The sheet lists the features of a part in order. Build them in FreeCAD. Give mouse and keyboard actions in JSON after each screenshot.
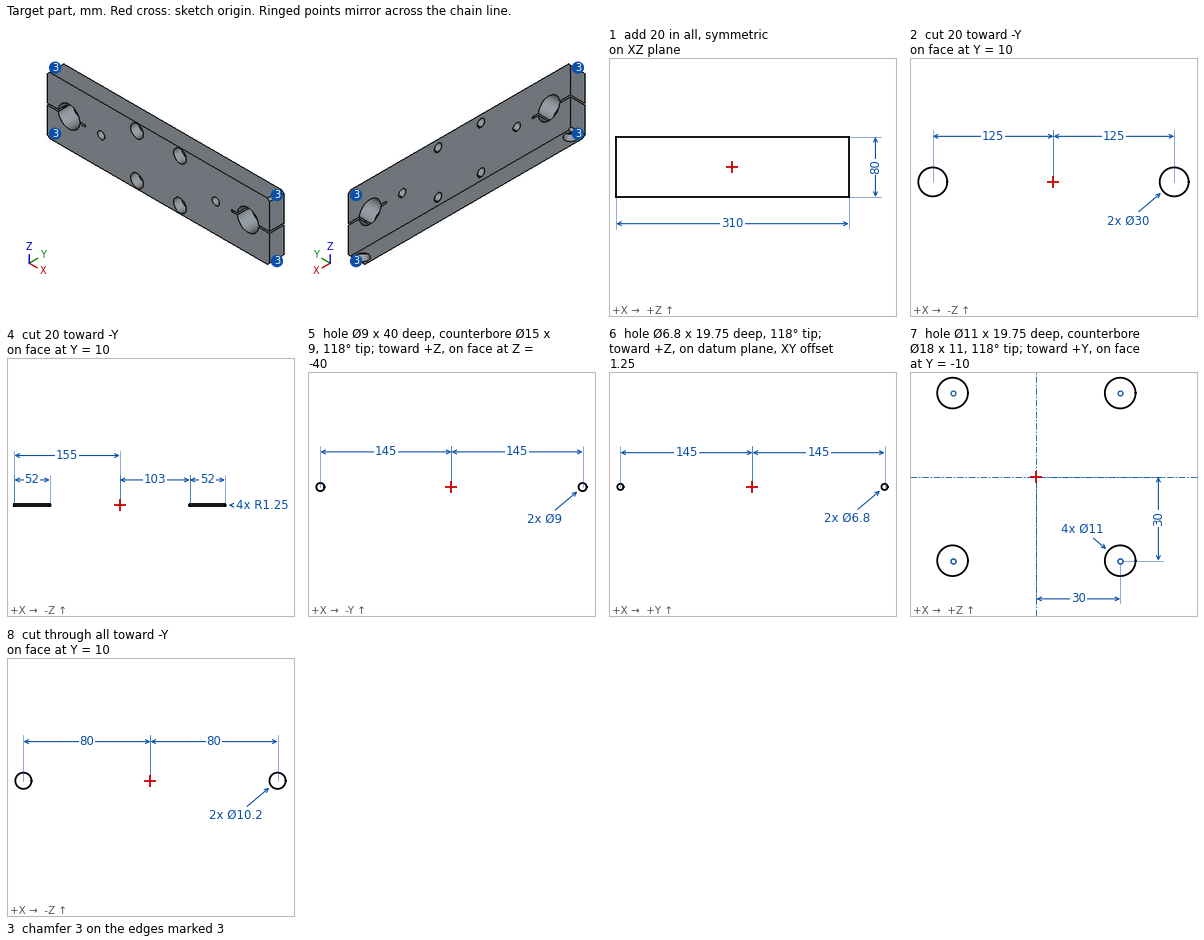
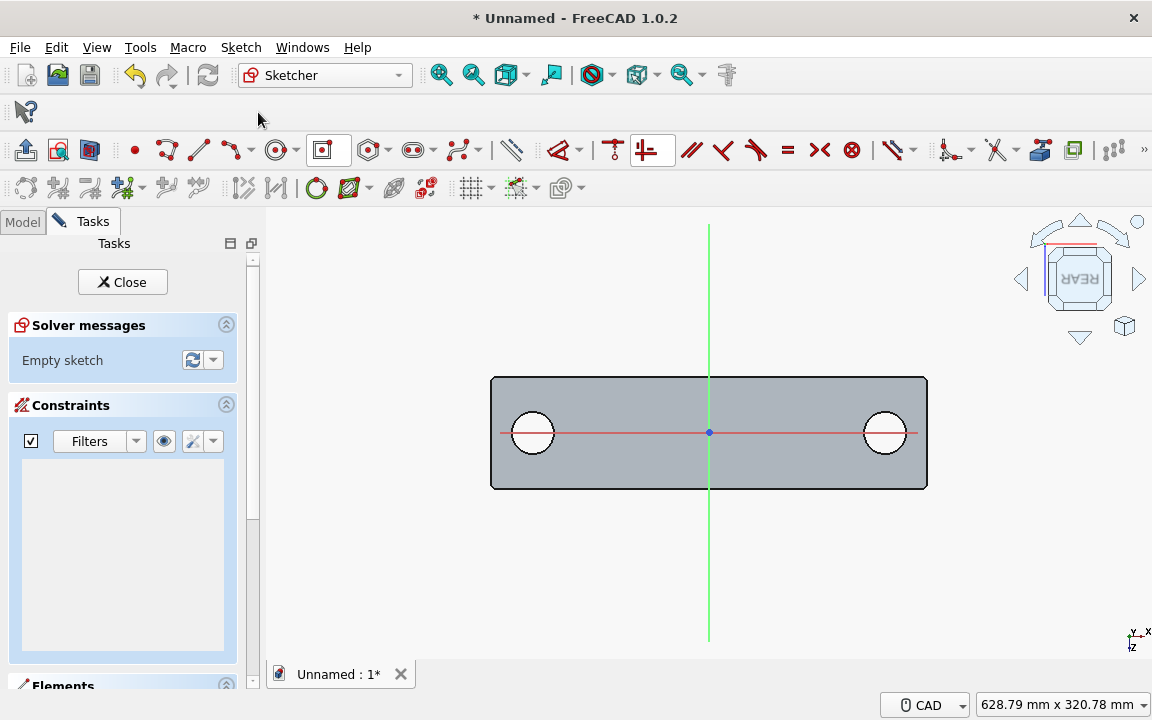
{"action": "left_click", "coordinate": [414, 150]}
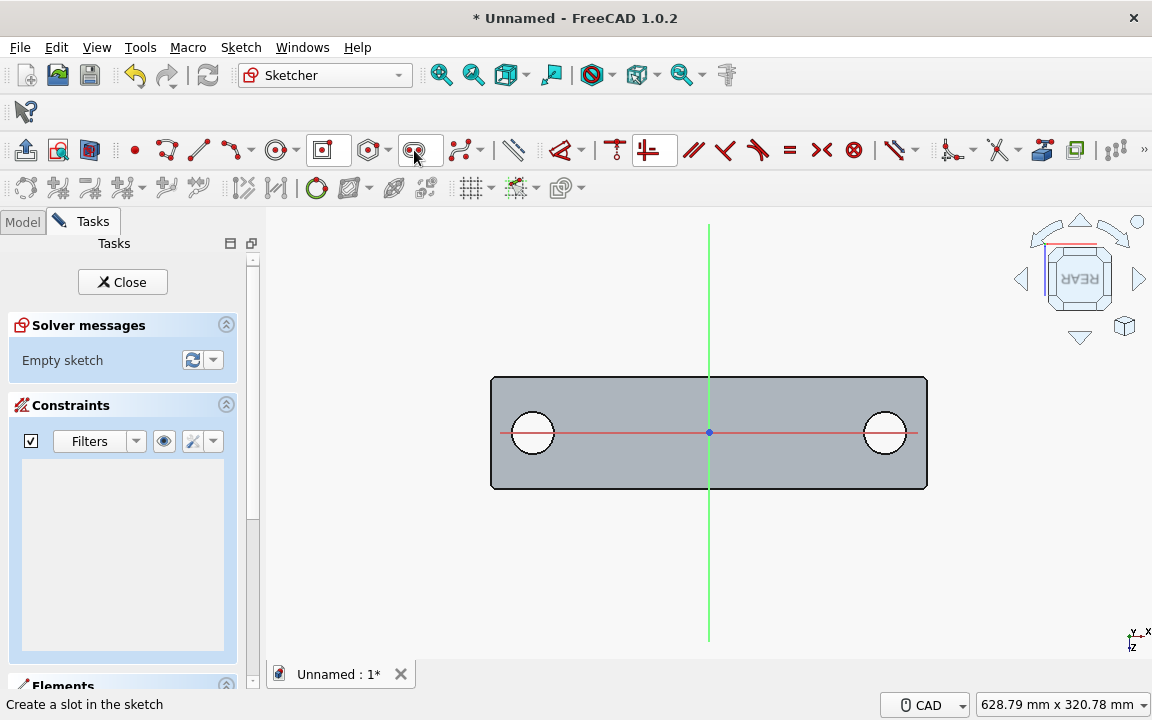
{"action": "scroll", "coordinate": [854, 433], "scroll_direction": "up", "scroll_amount": 13}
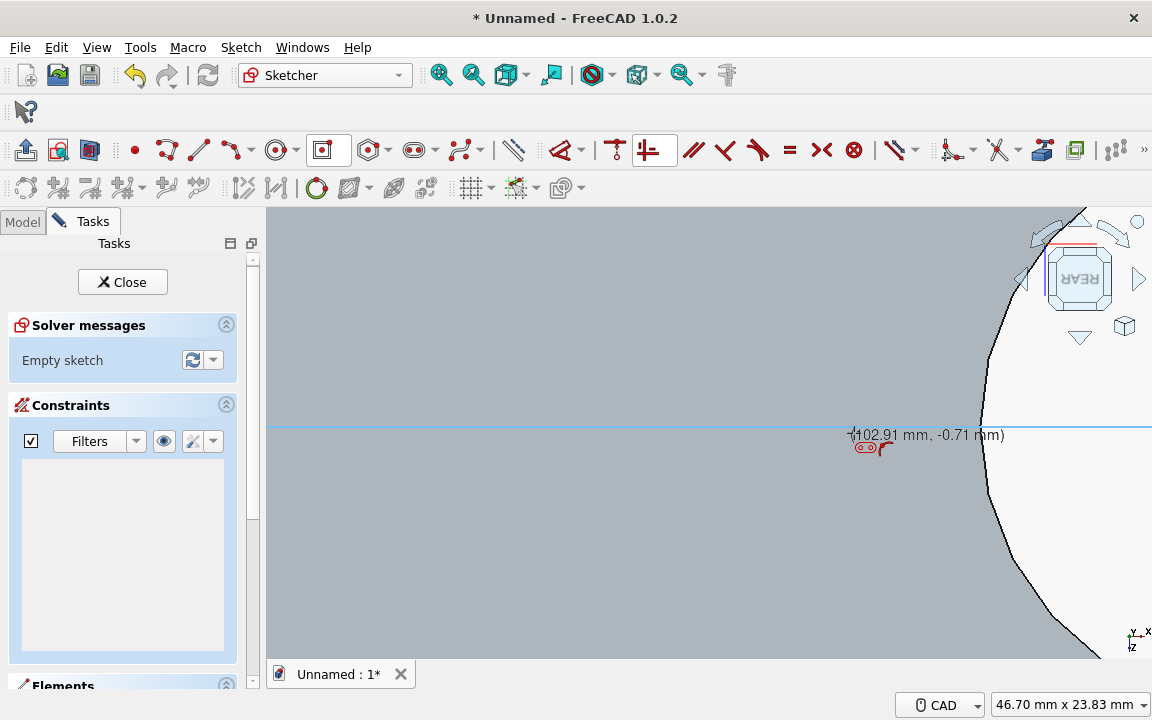
{"action": "scroll", "coordinate": [815, 434], "scroll_direction": "down", "scroll_amount": 12}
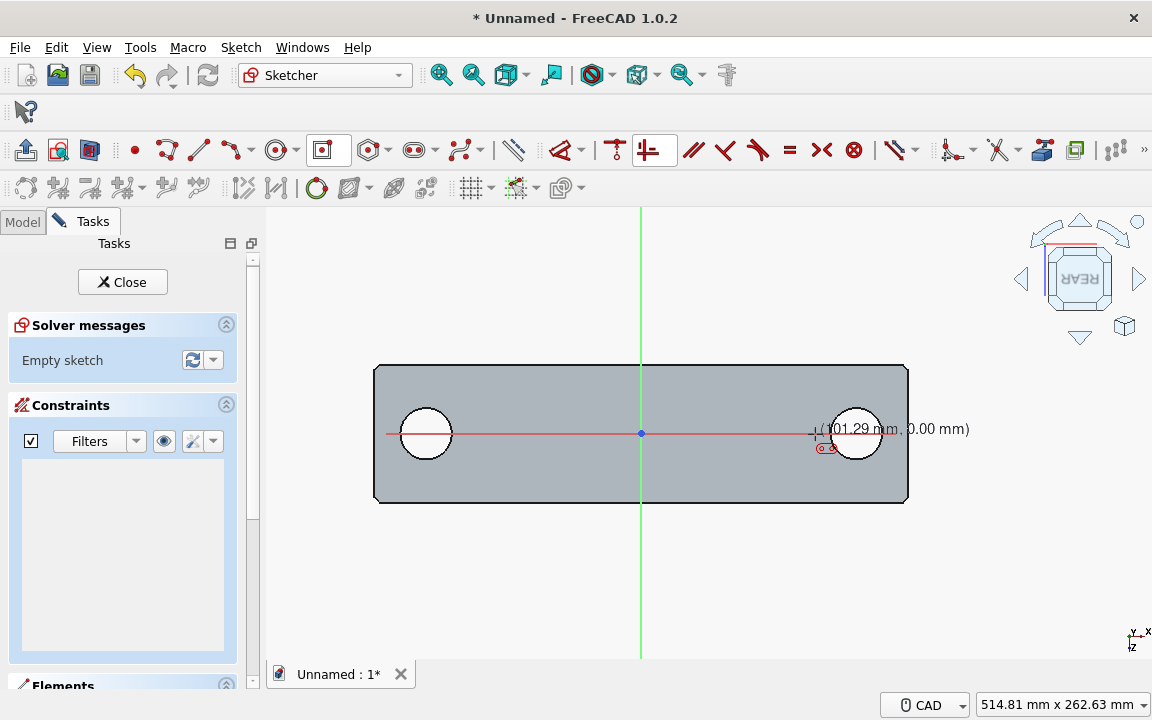
{"action": "left_click", "coordinate": [819, 434]}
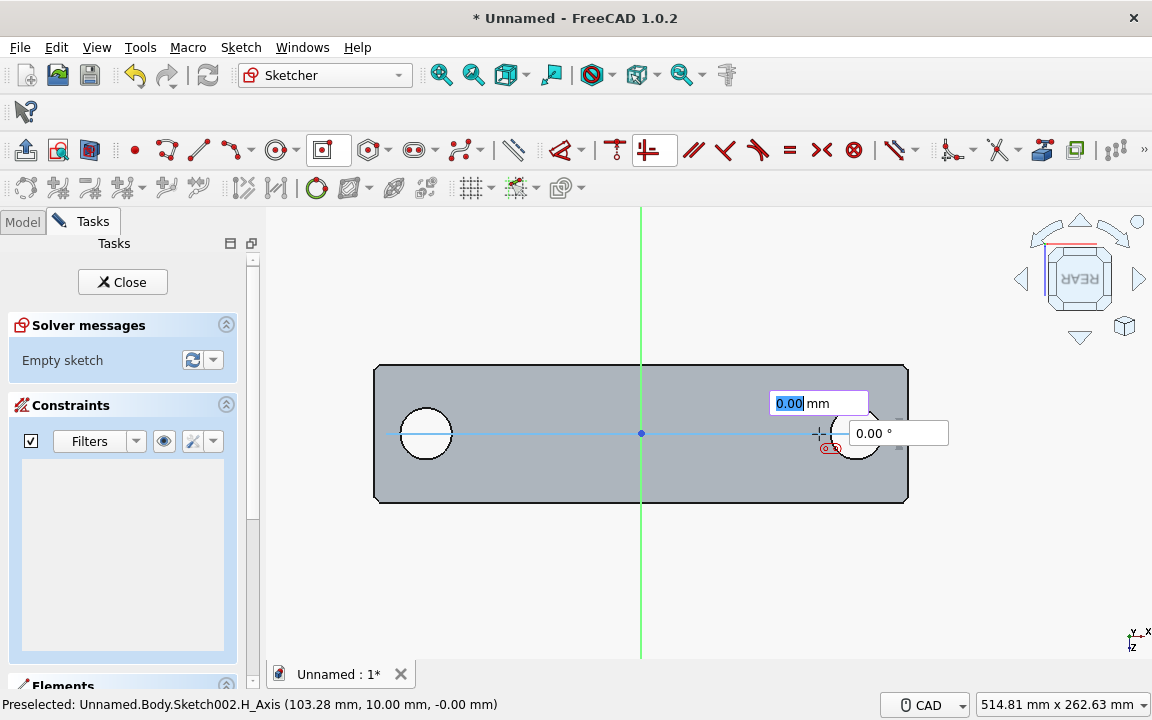
{"action": "left_click", "coordinate": [908, 425]}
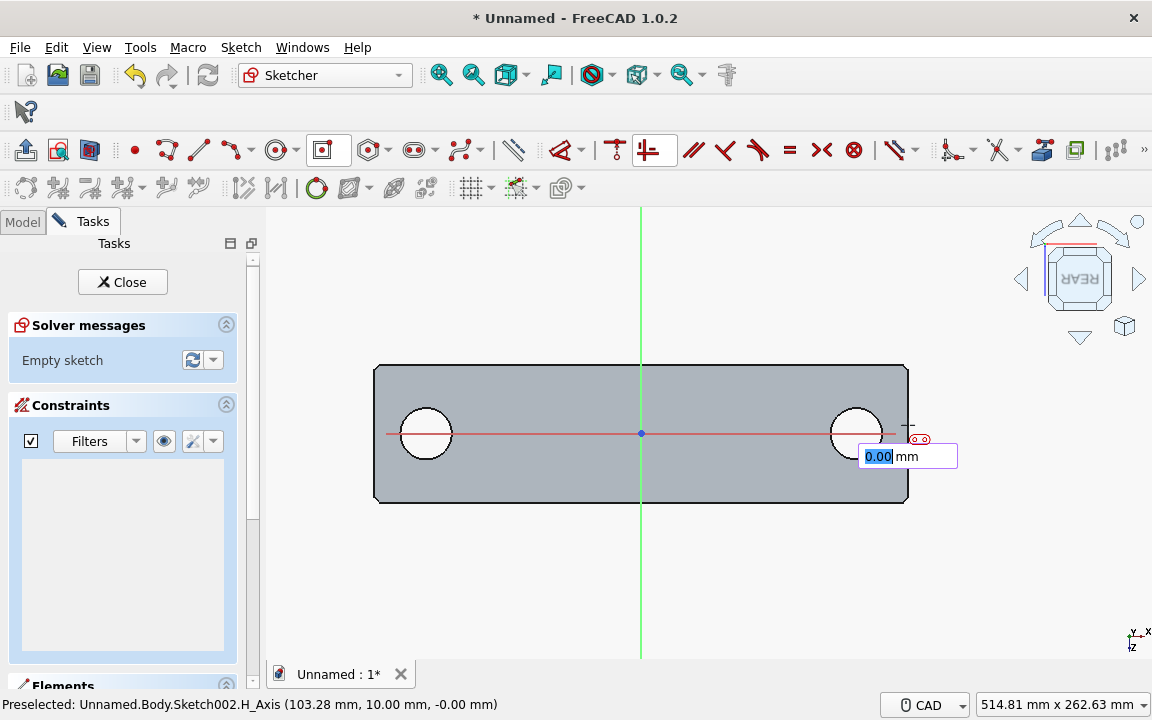
{"action": "scroll", "coordinate": [863, 436], "scroll_direction": "up", "scroll_amount": 10}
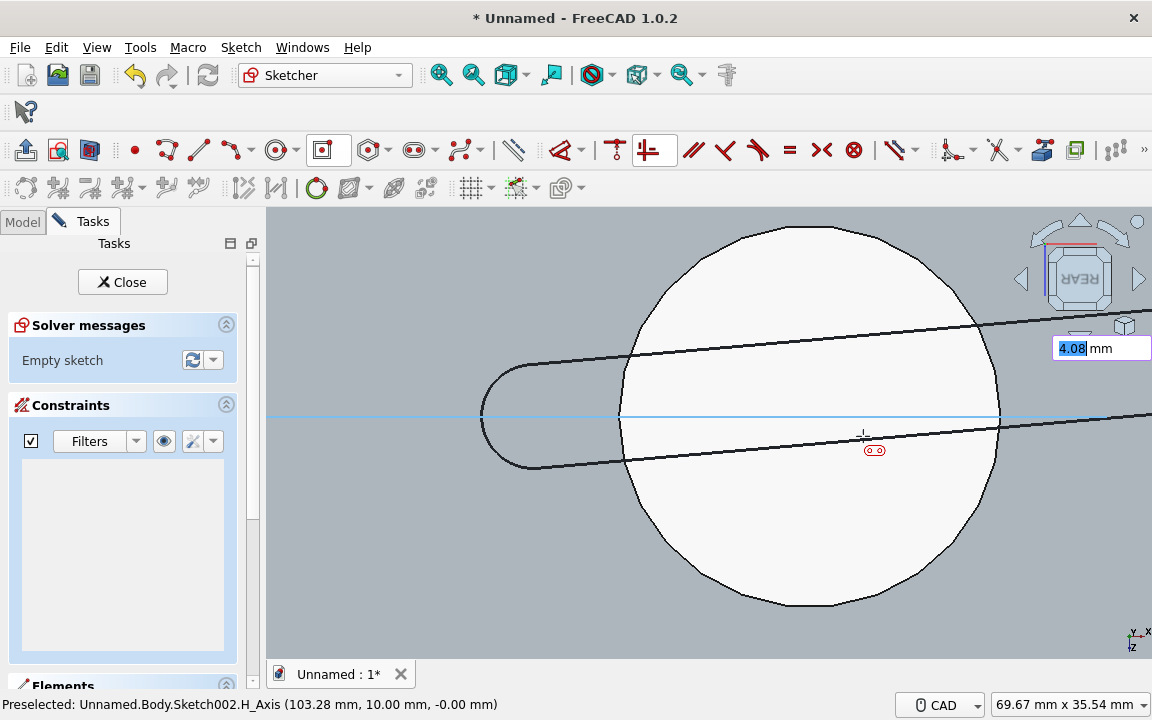
{"action": "left_click", "coordinate": [861, 432]}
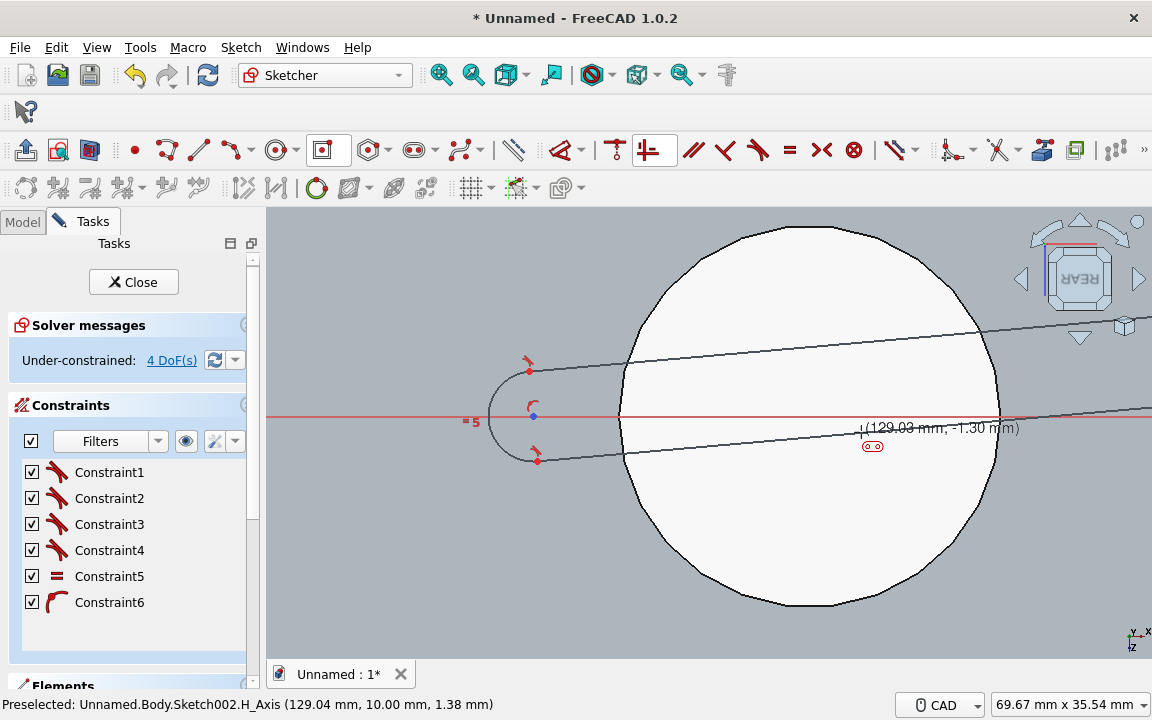
{"action": "scroll", "coordinate": [863, 436], "scroll_direction": "down", "scroll_amount": 10}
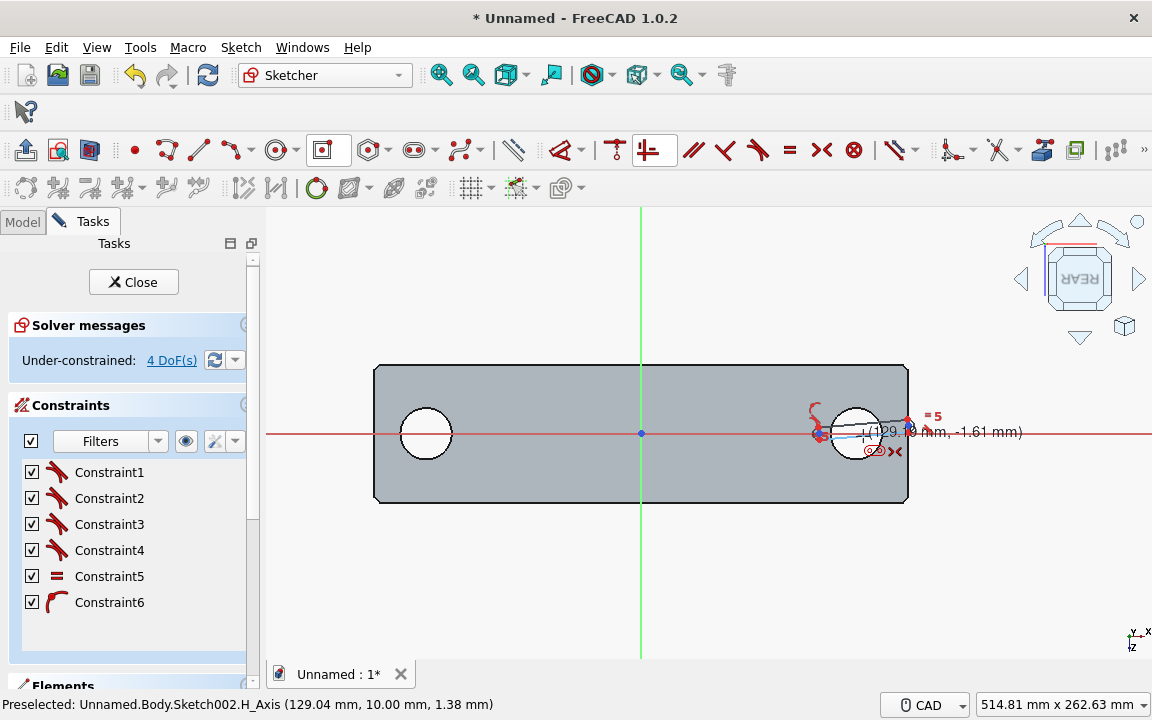
{"action": "scroll", "coordinate": [374, 434], "scroll_direction": "up", "scroll_amount": 12}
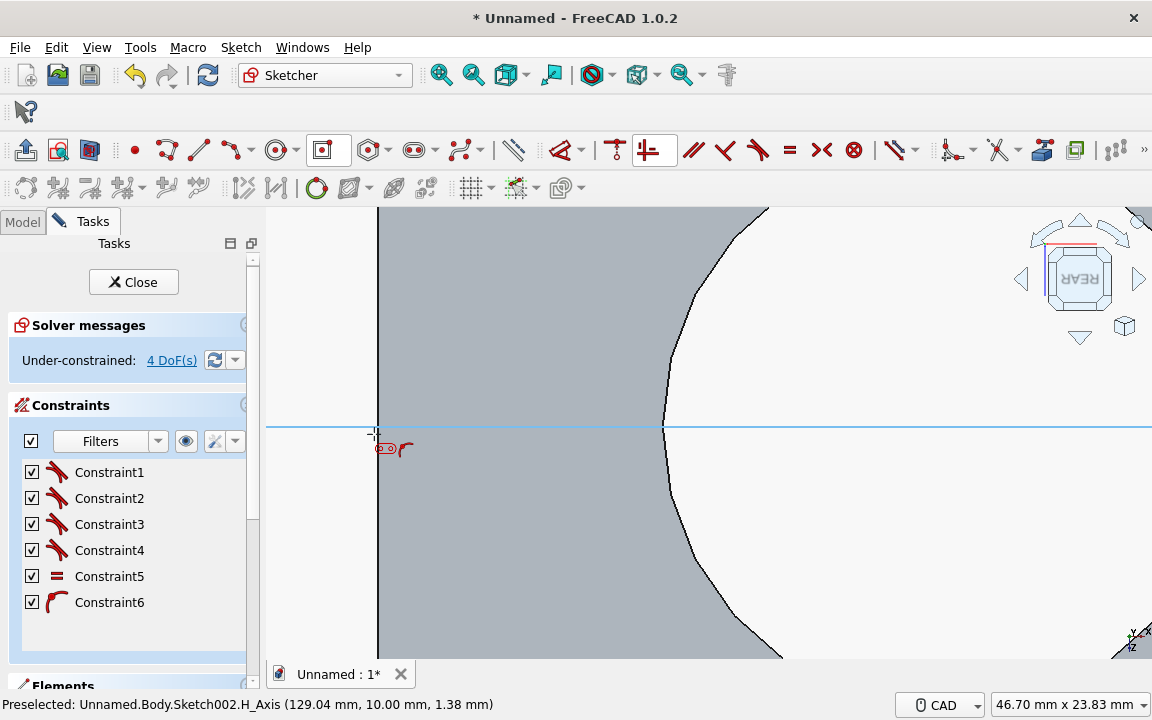
{"action": "scroll", "coordinate": [373, 434], "scroll_direction": "down", "scroll_amount": 12}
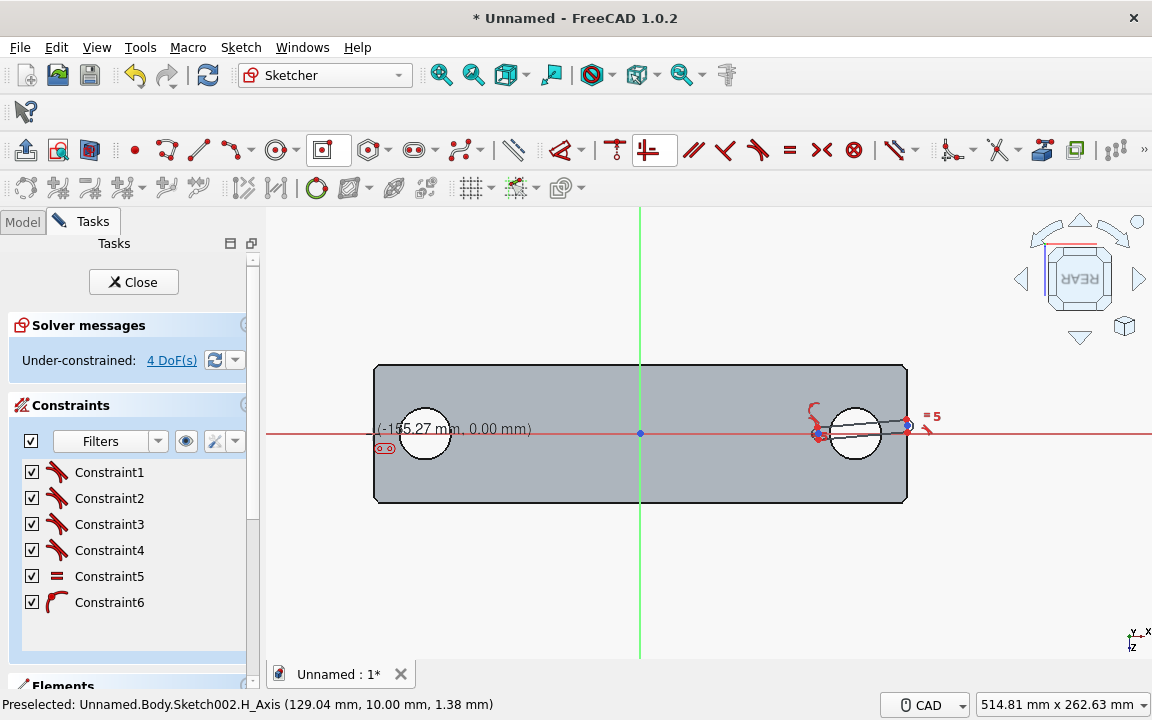
{"action": "left_click", "coordinate": [374, 434]}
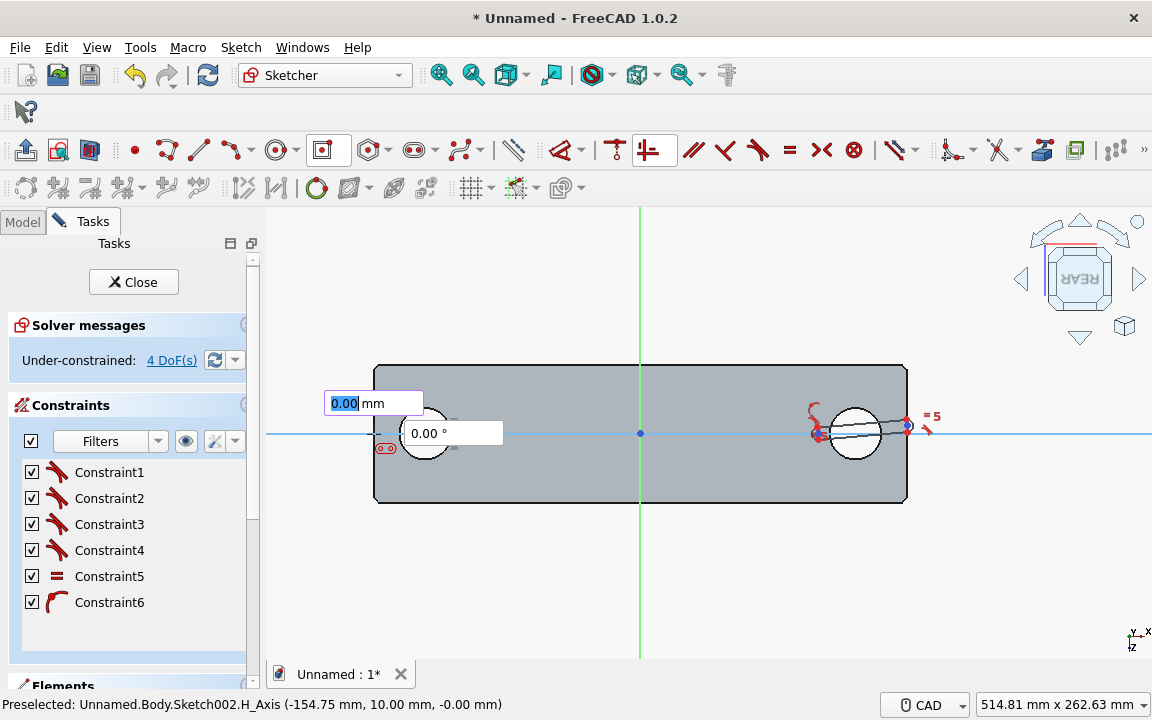
{"action": "left_click", "coordinate": [463, 425]}